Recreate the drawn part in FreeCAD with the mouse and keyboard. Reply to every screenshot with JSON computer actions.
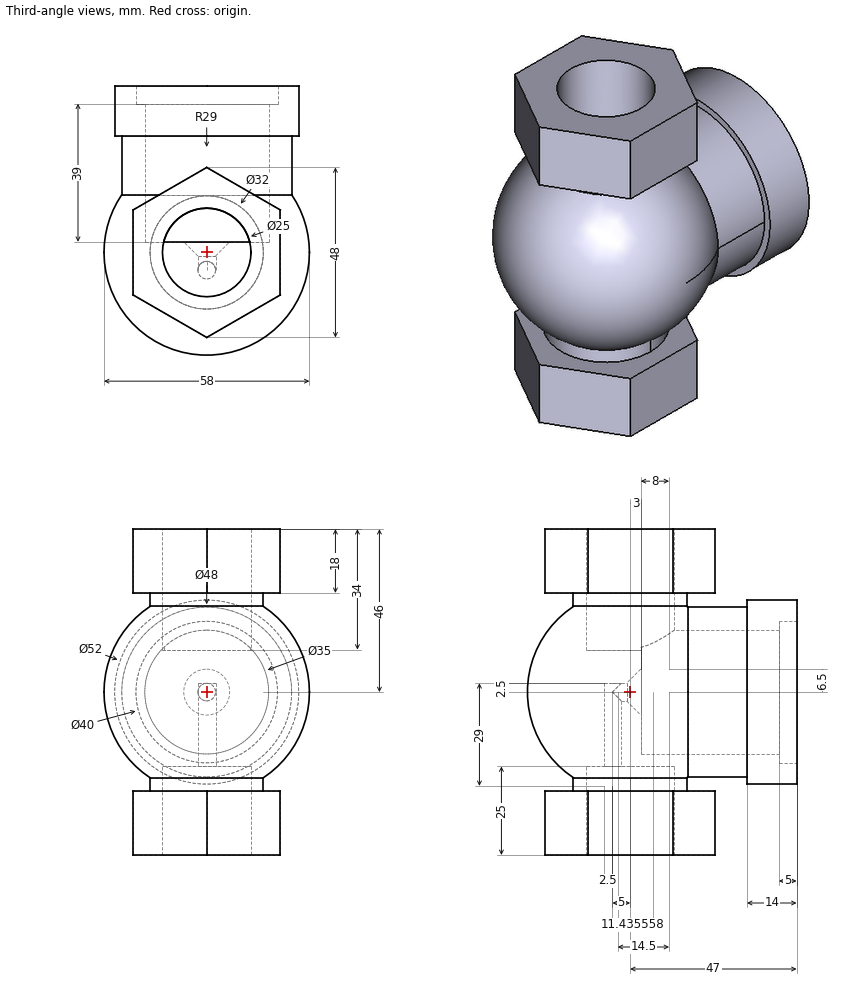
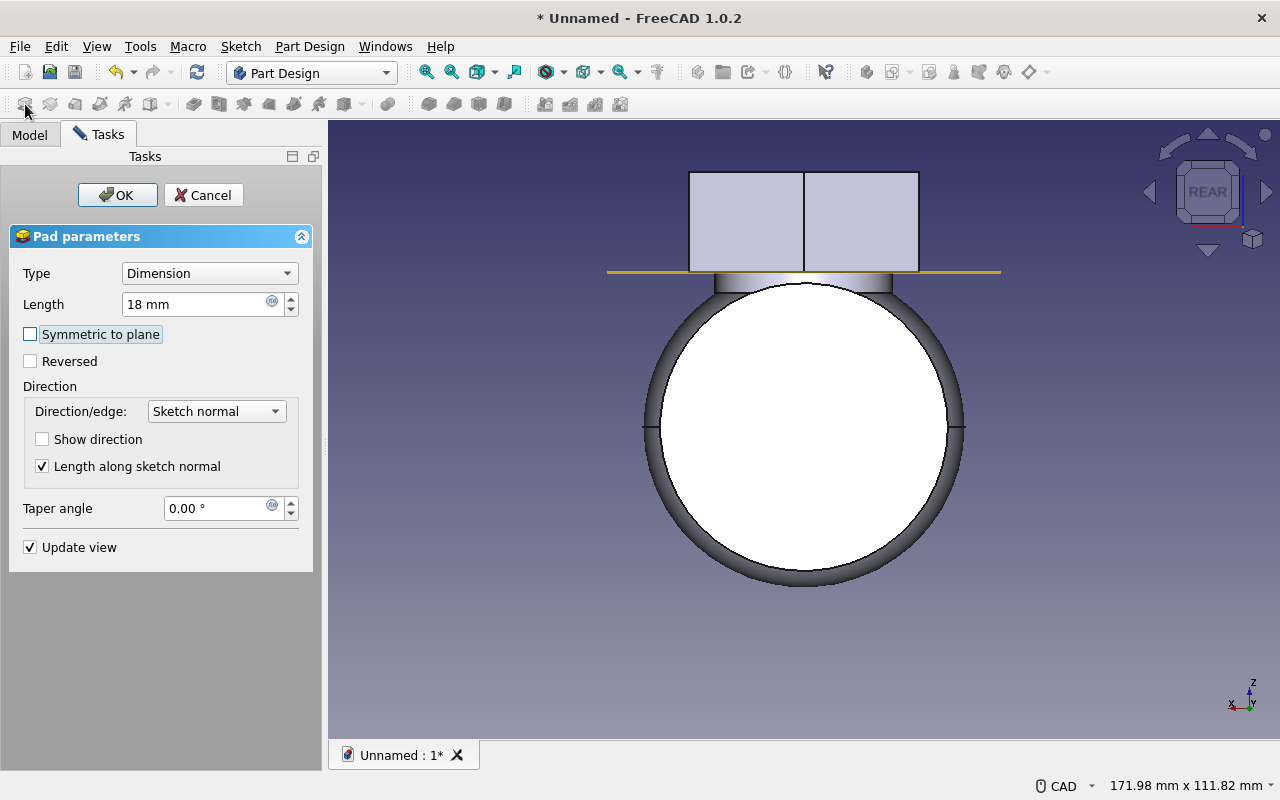
{"action": "left_click", "coordinate": [118, 195]}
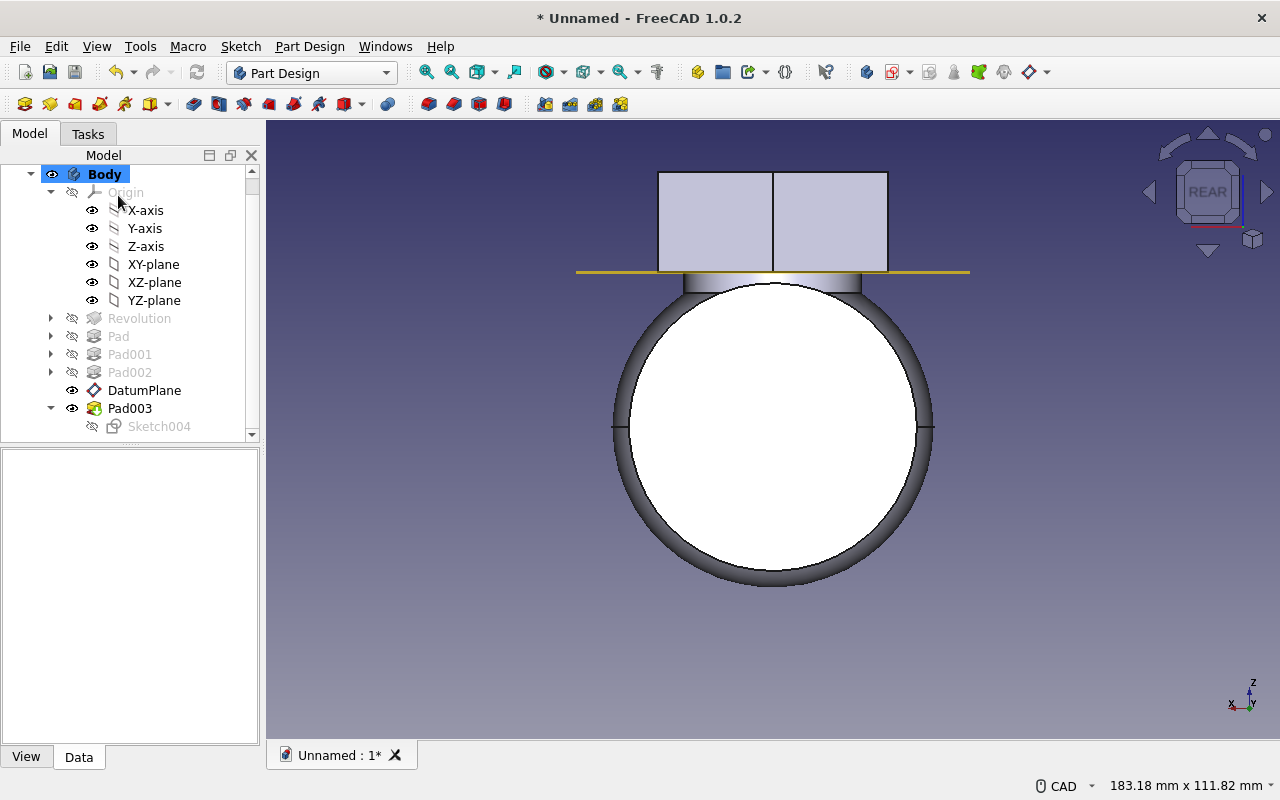
{"action": "left_click", "coordinate": [117, 390]}
{"action": "key", "text": "space"}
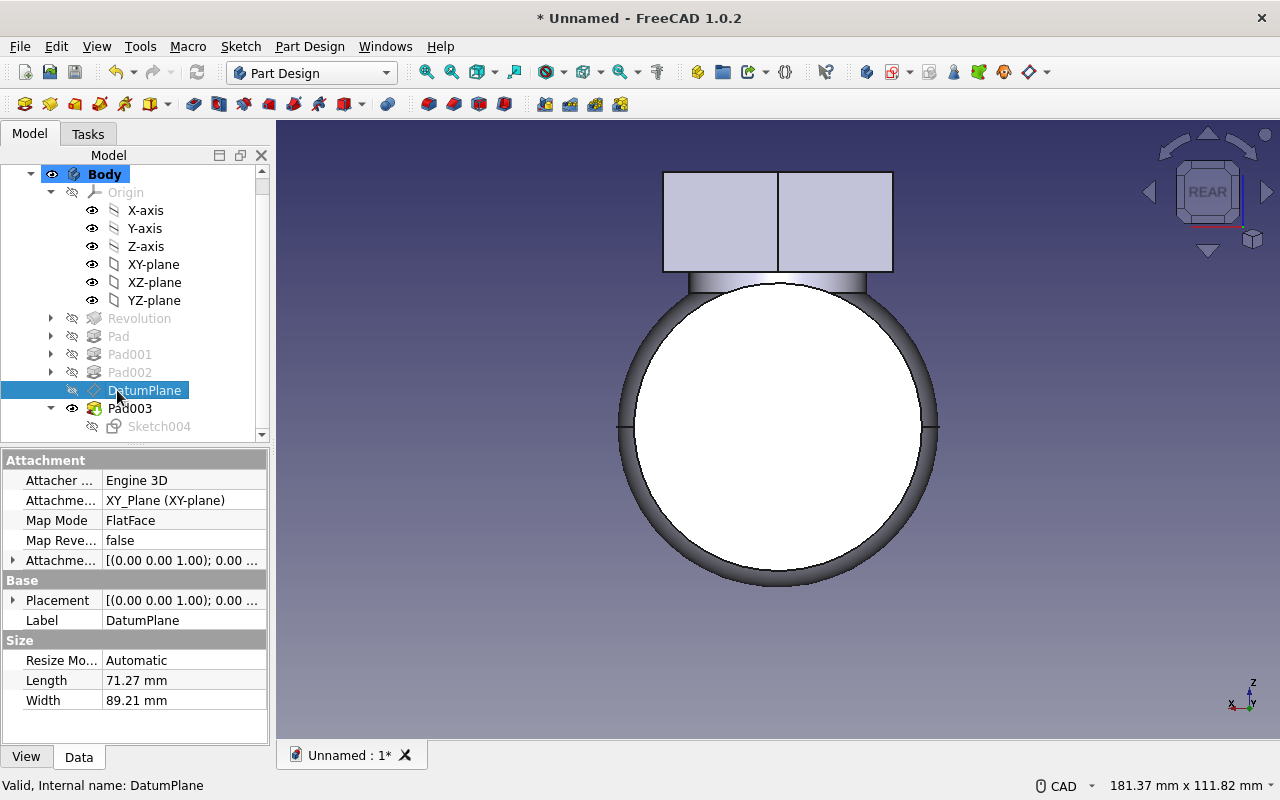
{"action": "left_click", "coordinate": [778, 426]}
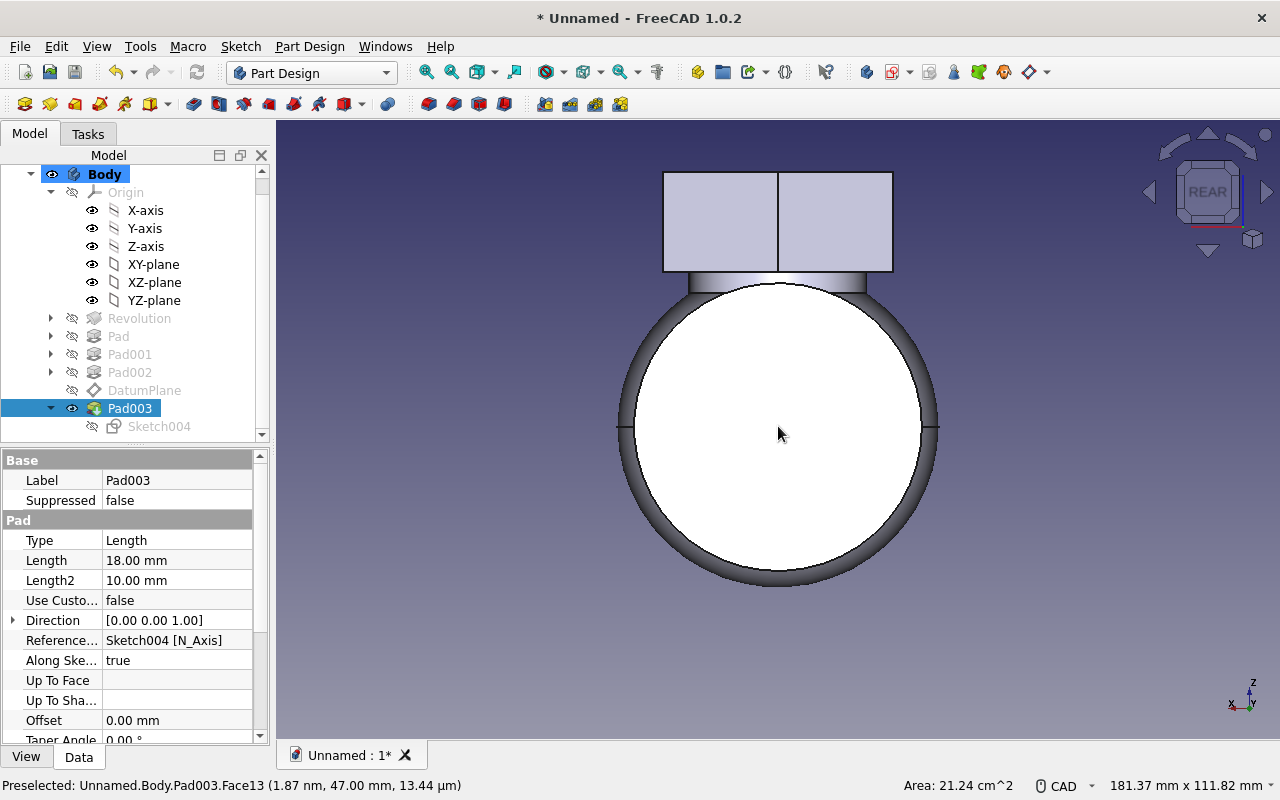
{"action": "left_click", "coordinate": [892, 72]}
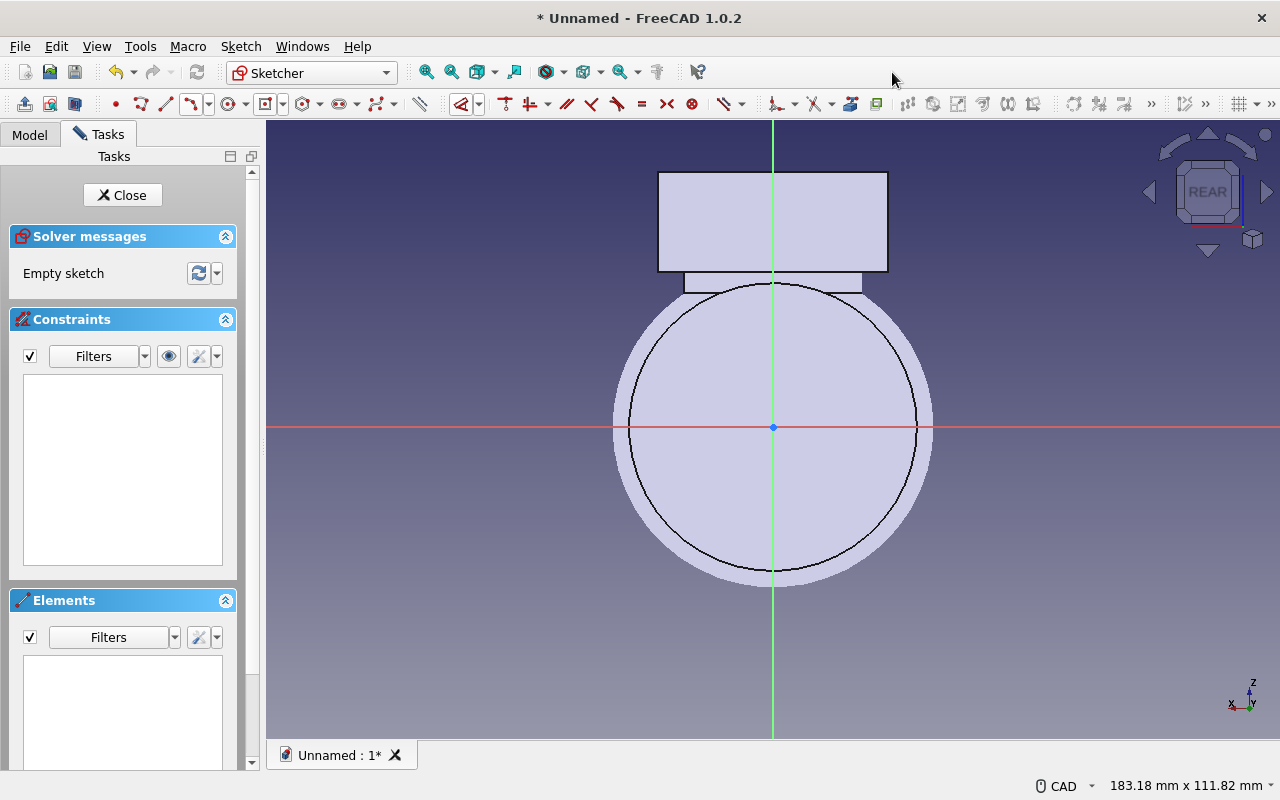
{"action": "scroll", "coordinate": [856, 424], "scroll_direction": "up", "scroll_amount": 3}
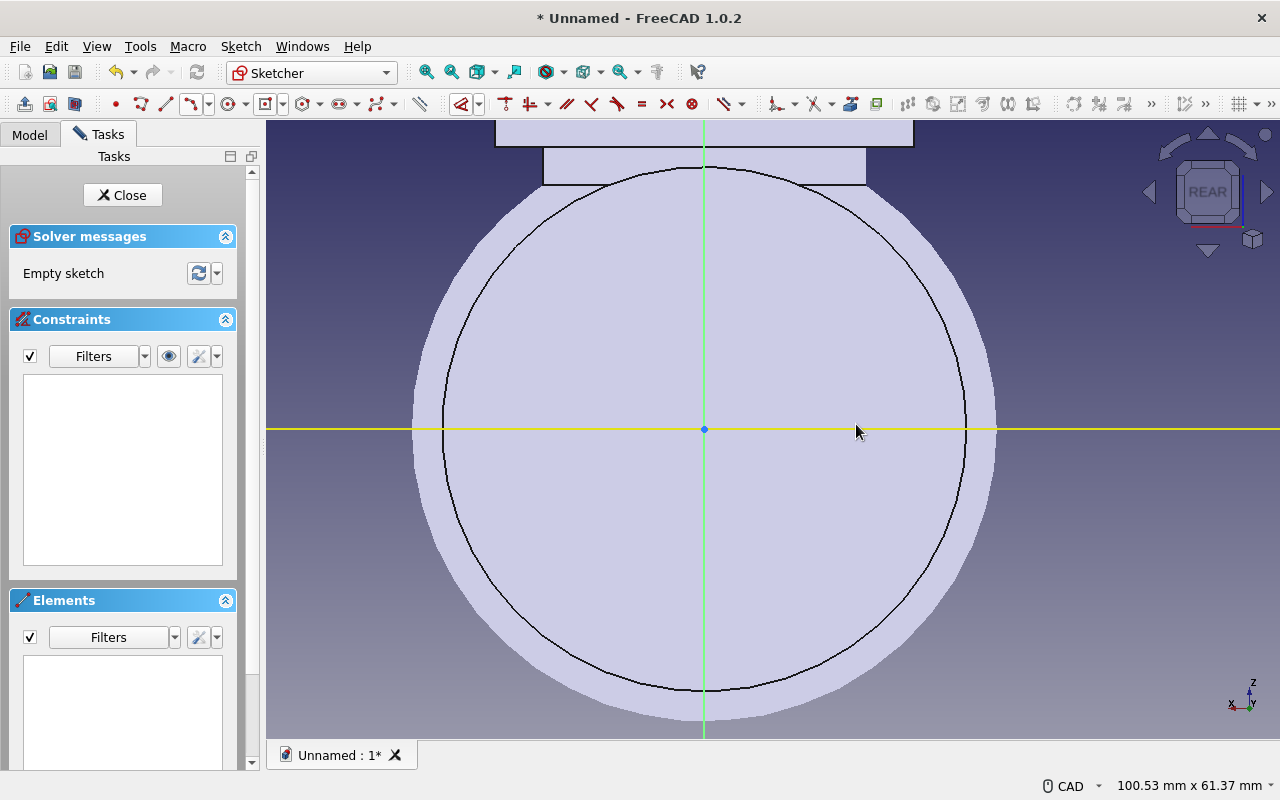
{"action": "key", "text": "g c"}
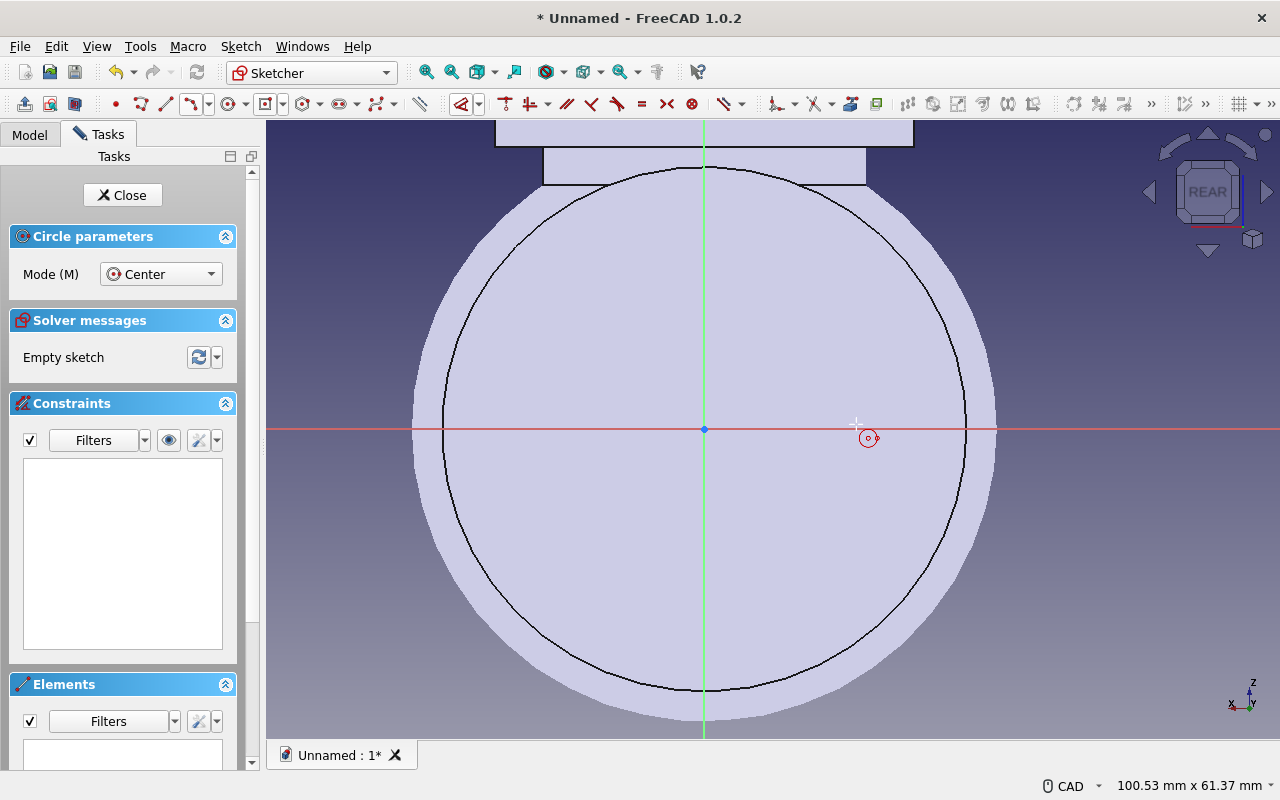
{"action": "left_click", "coordinate": [704, 429]}
{"action": "left_click", "coordinate": [847, 287]}
{"action": "key", "text": "Escape"}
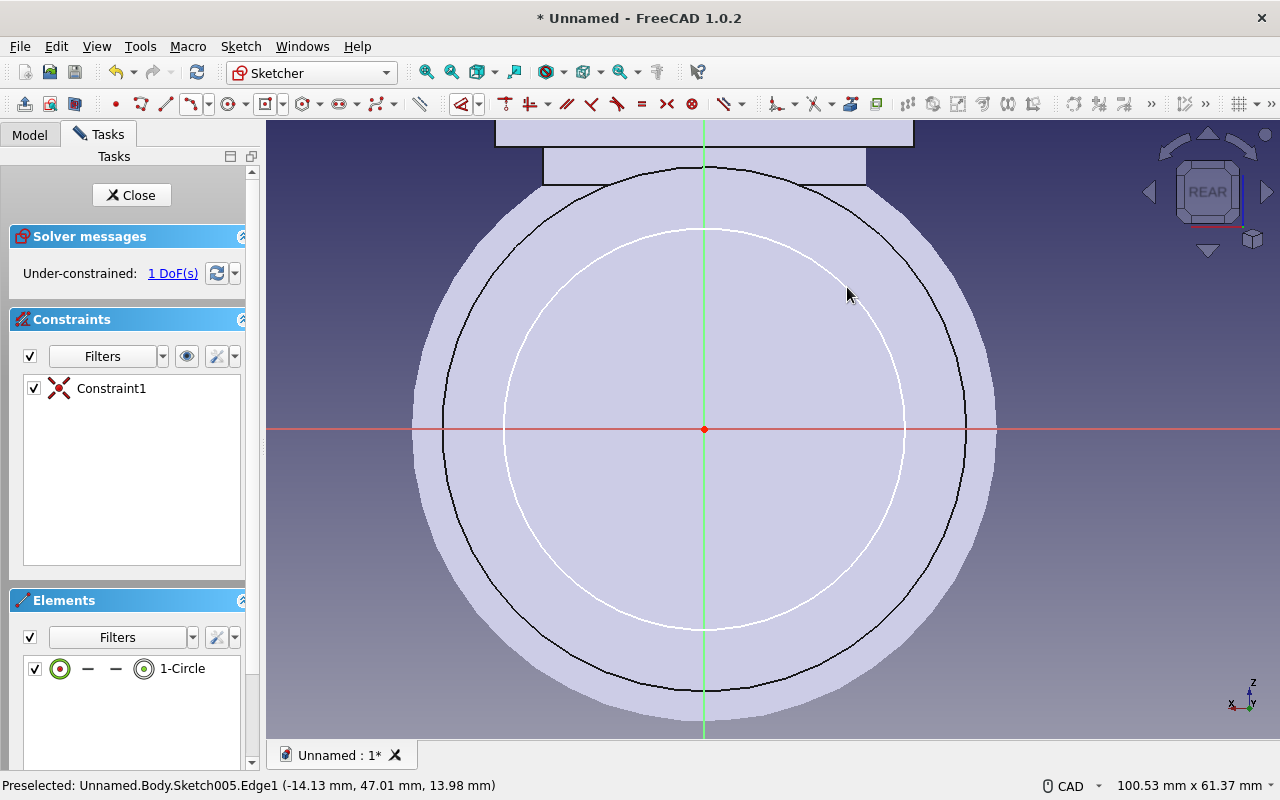
{"action": "left_click", "coordinate": [846, 287]}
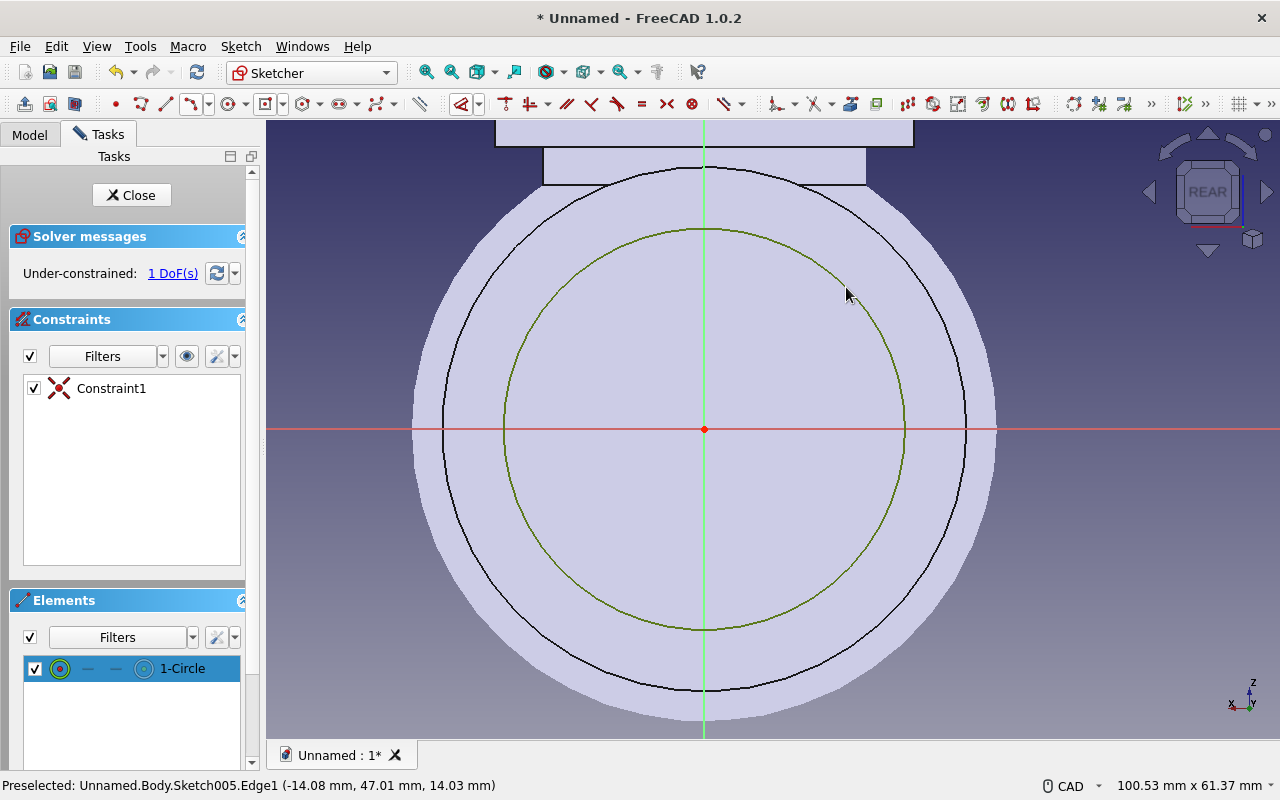
{"action": "key", "text": "k o"}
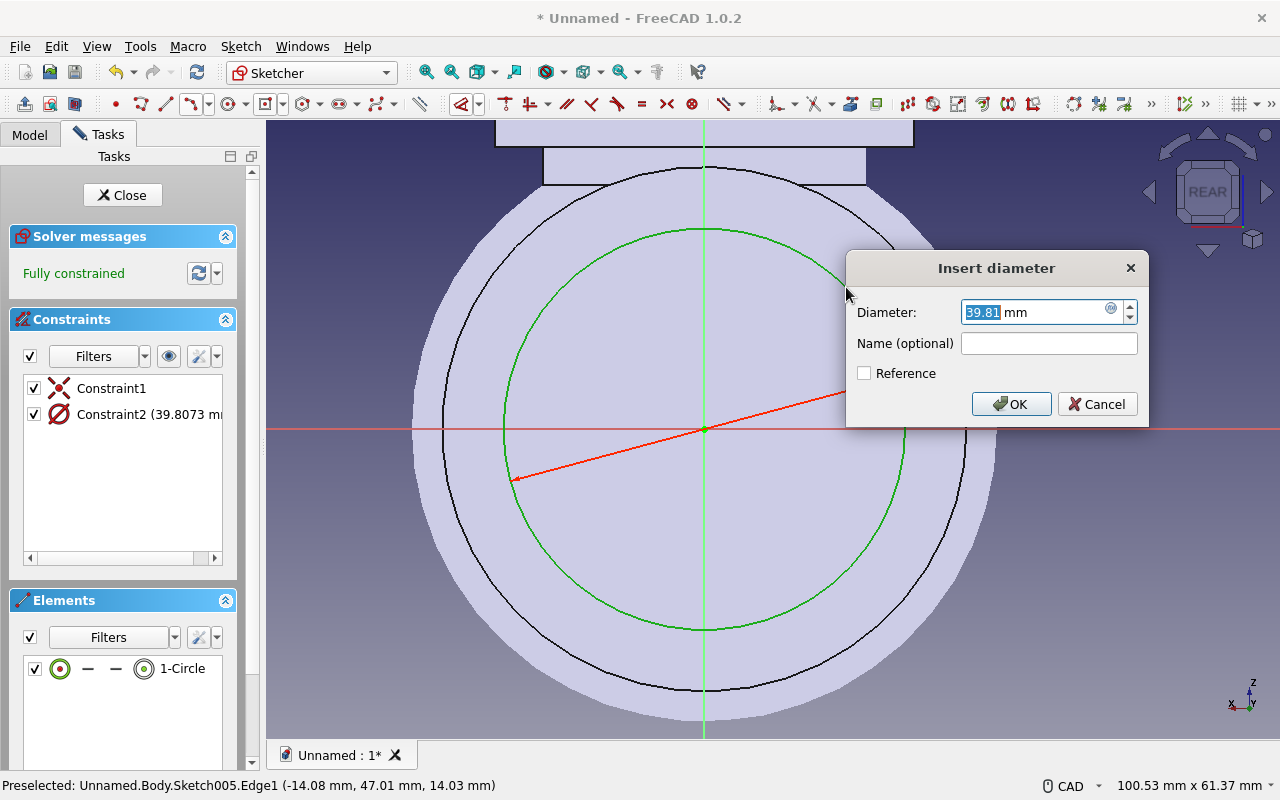
{"action": "type", "text": "40"}
{"action": "key", "text": "Return"}